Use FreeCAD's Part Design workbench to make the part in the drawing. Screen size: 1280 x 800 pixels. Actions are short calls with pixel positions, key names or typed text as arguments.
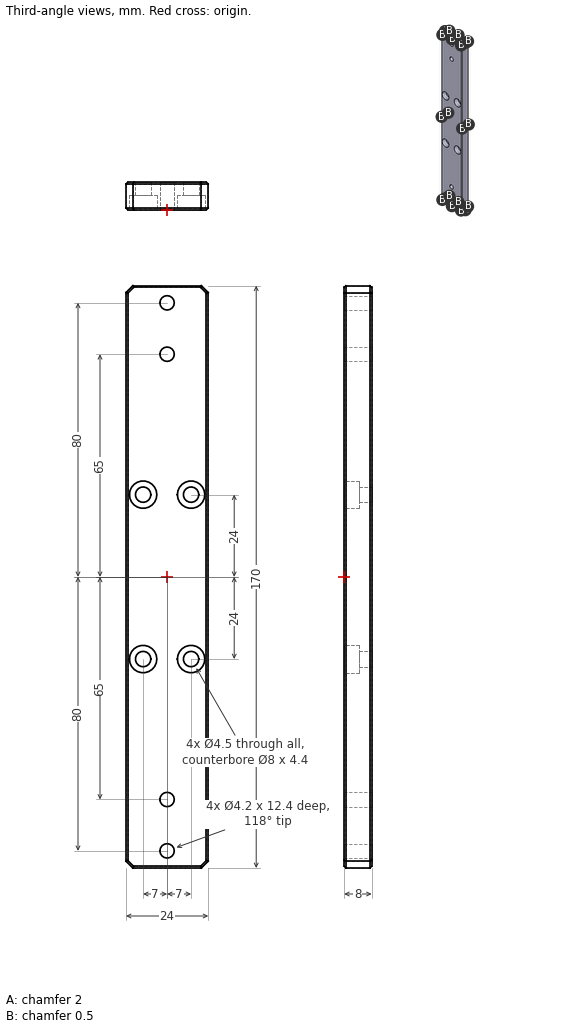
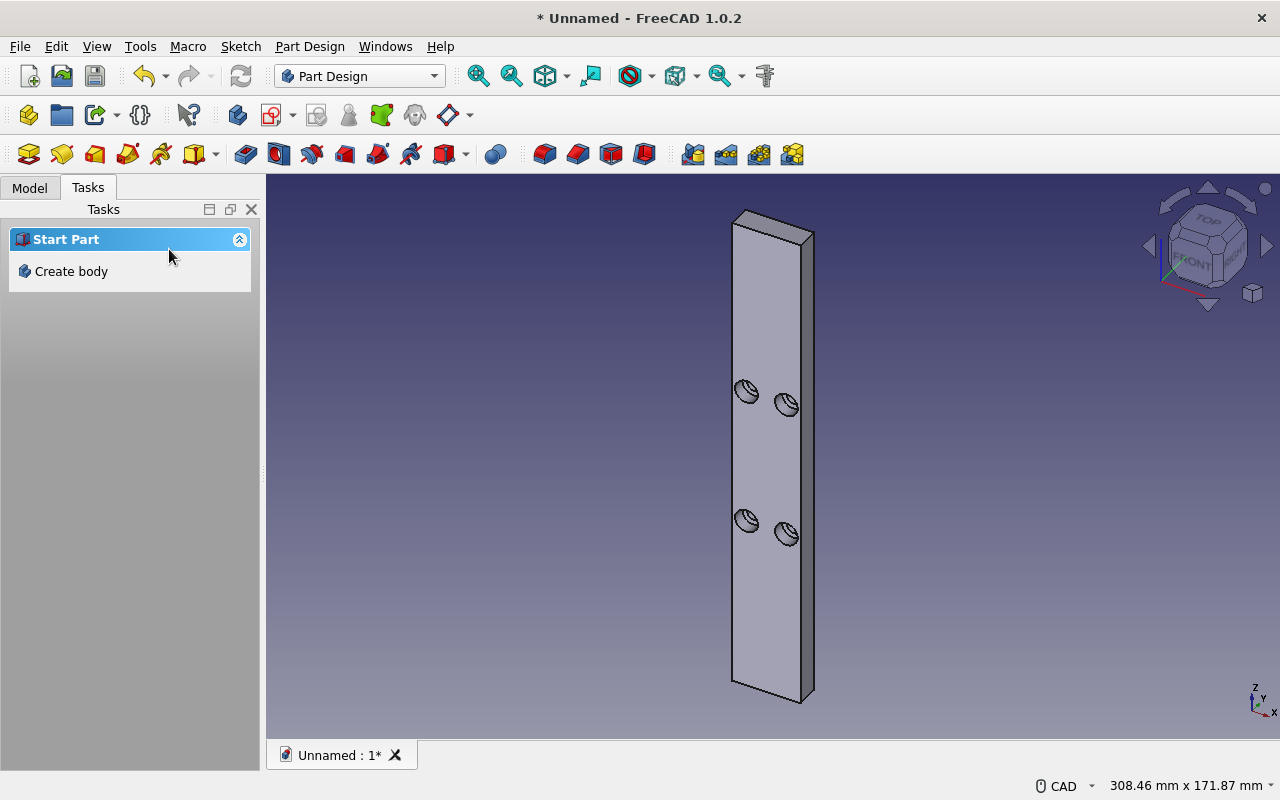
key(4)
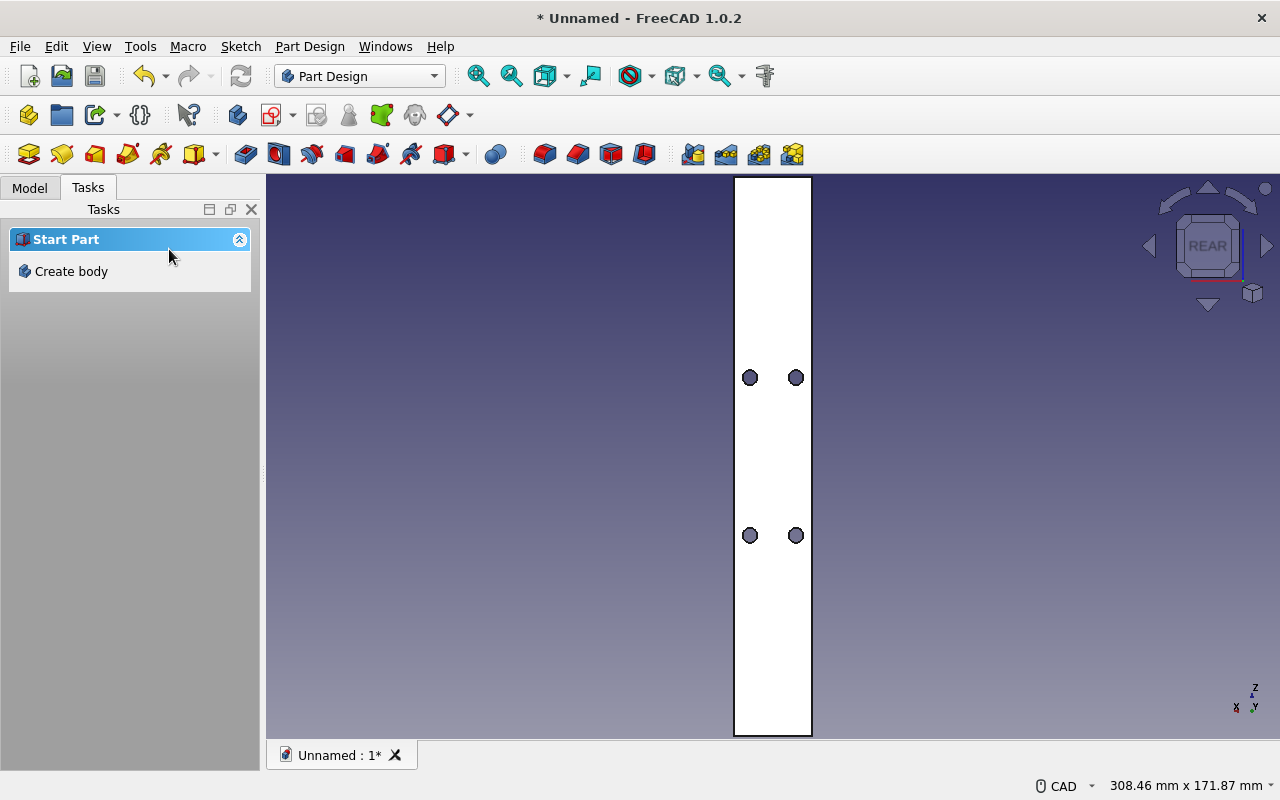
click(773, 216)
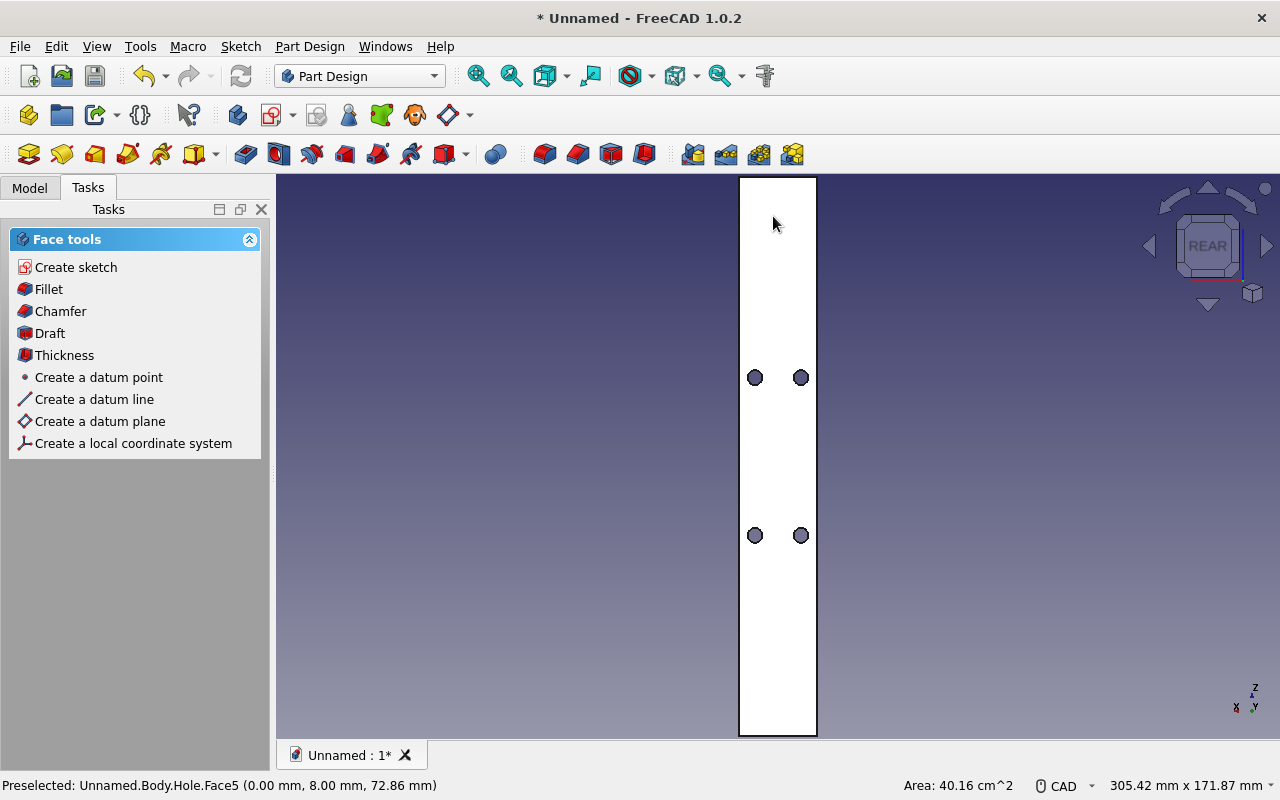
click(270, 116)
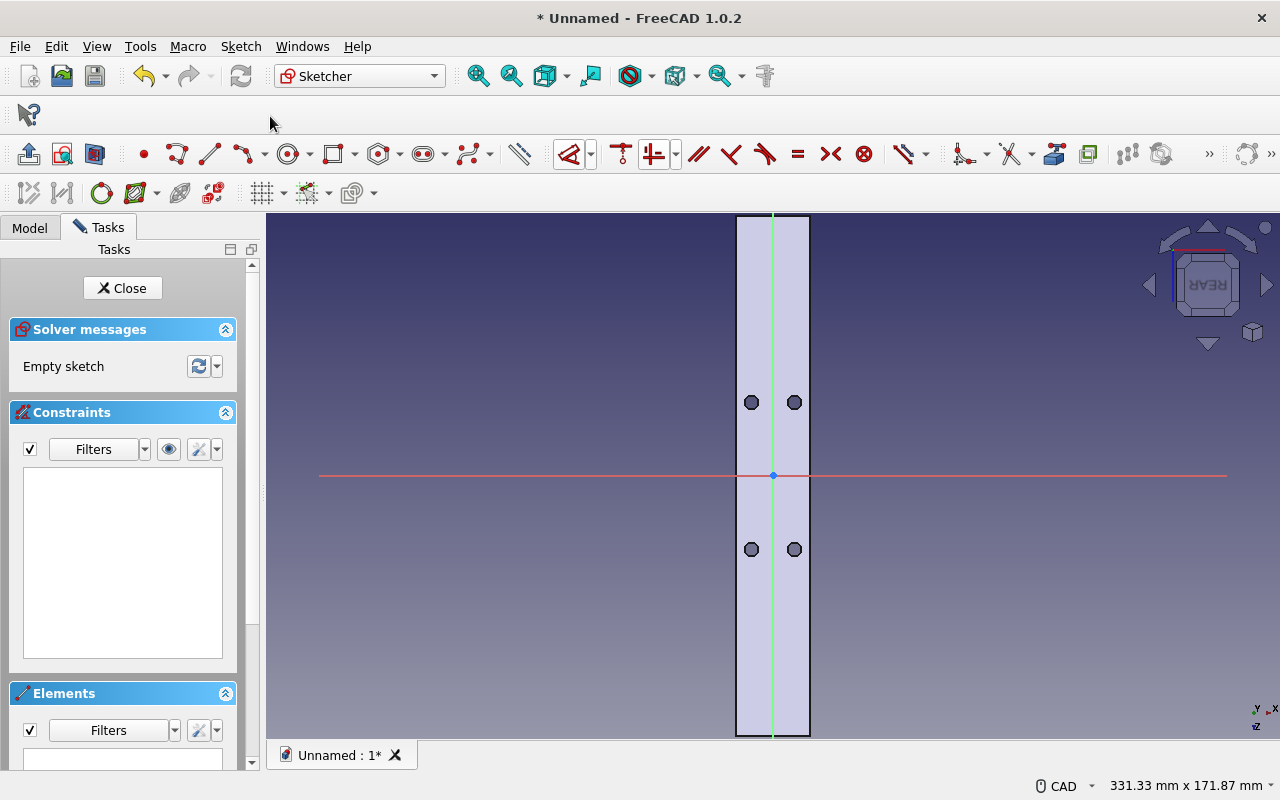
scroll(565, 476, down, 2)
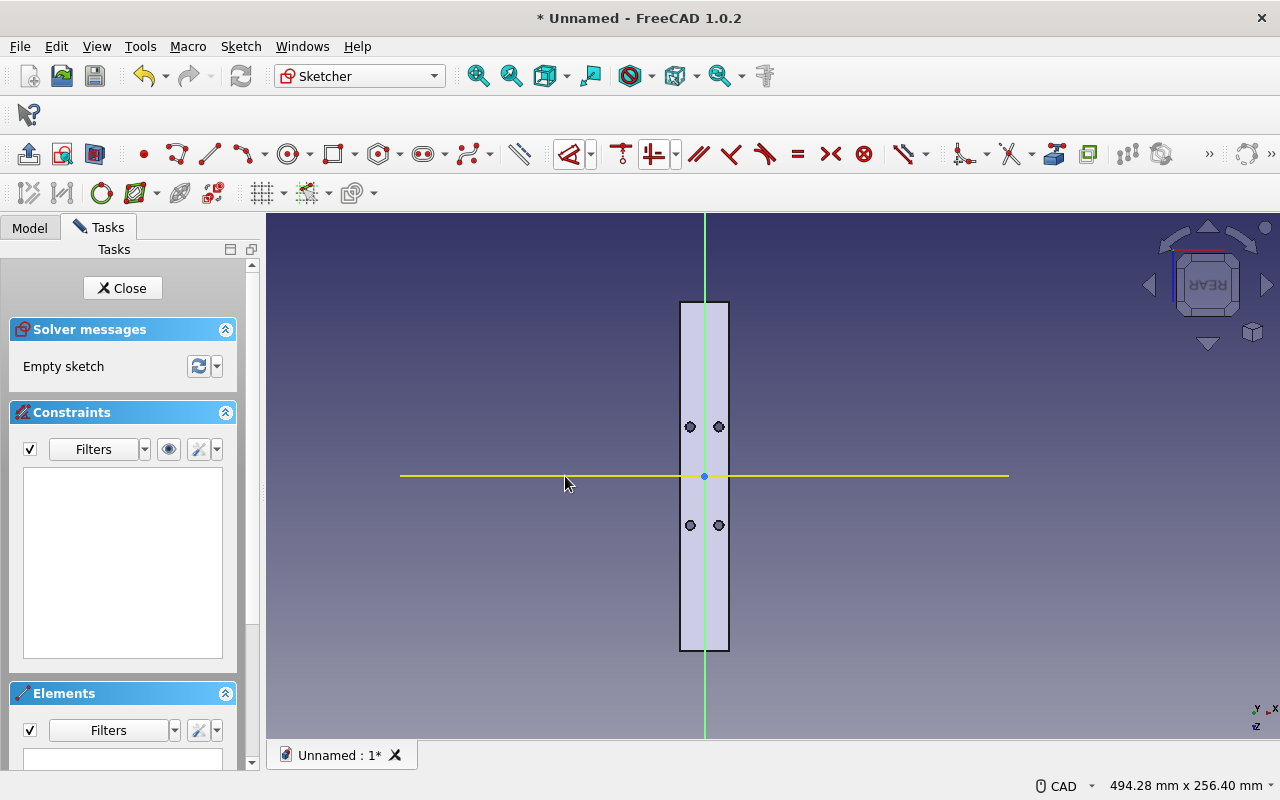
click(288, 154)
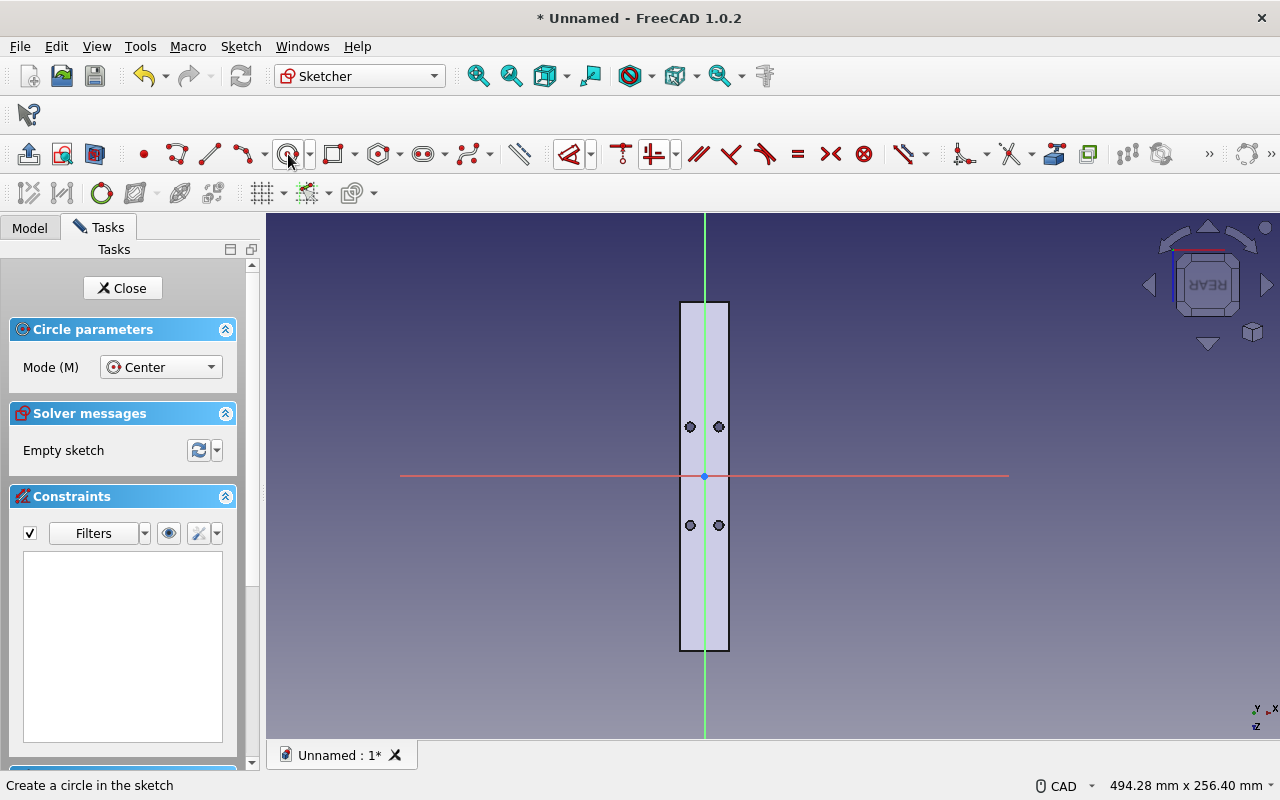
scroll(705, 312, up, 9)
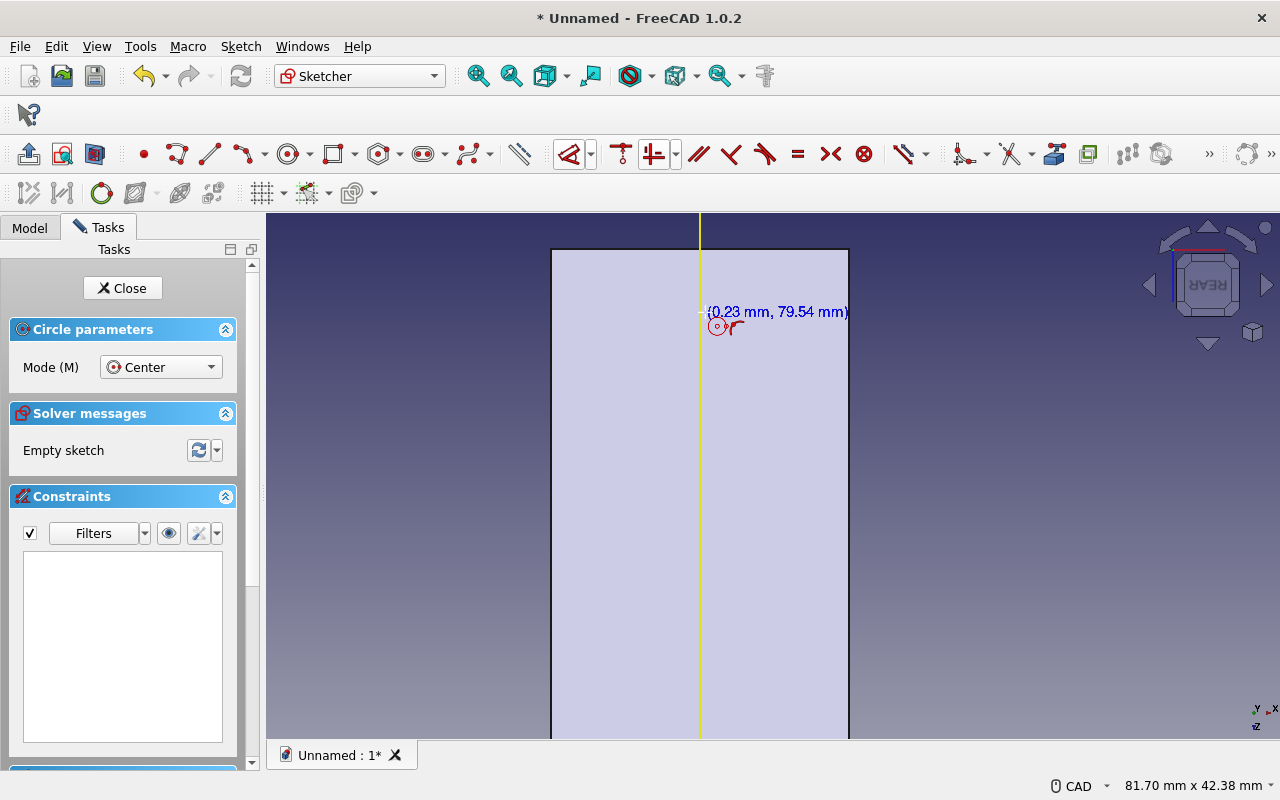
scroll(705, 312, down, 9)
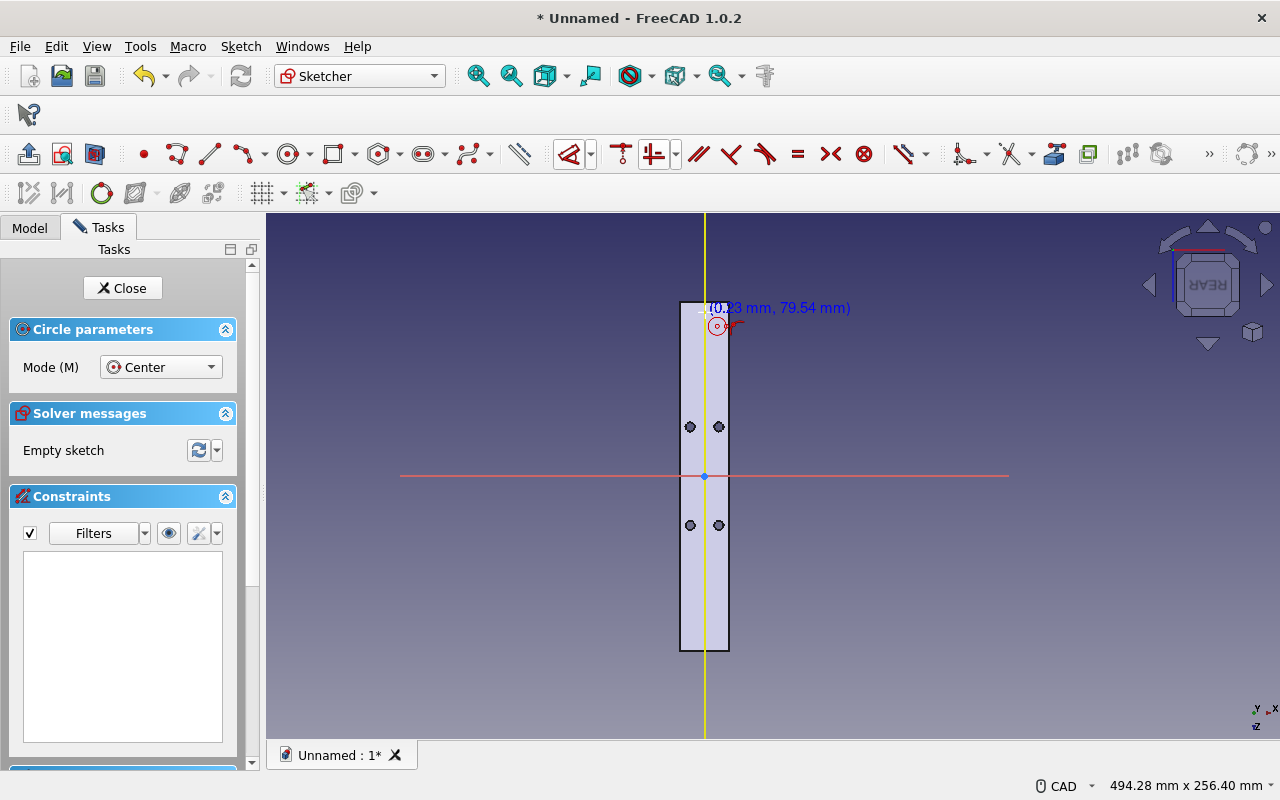
click(705, 312)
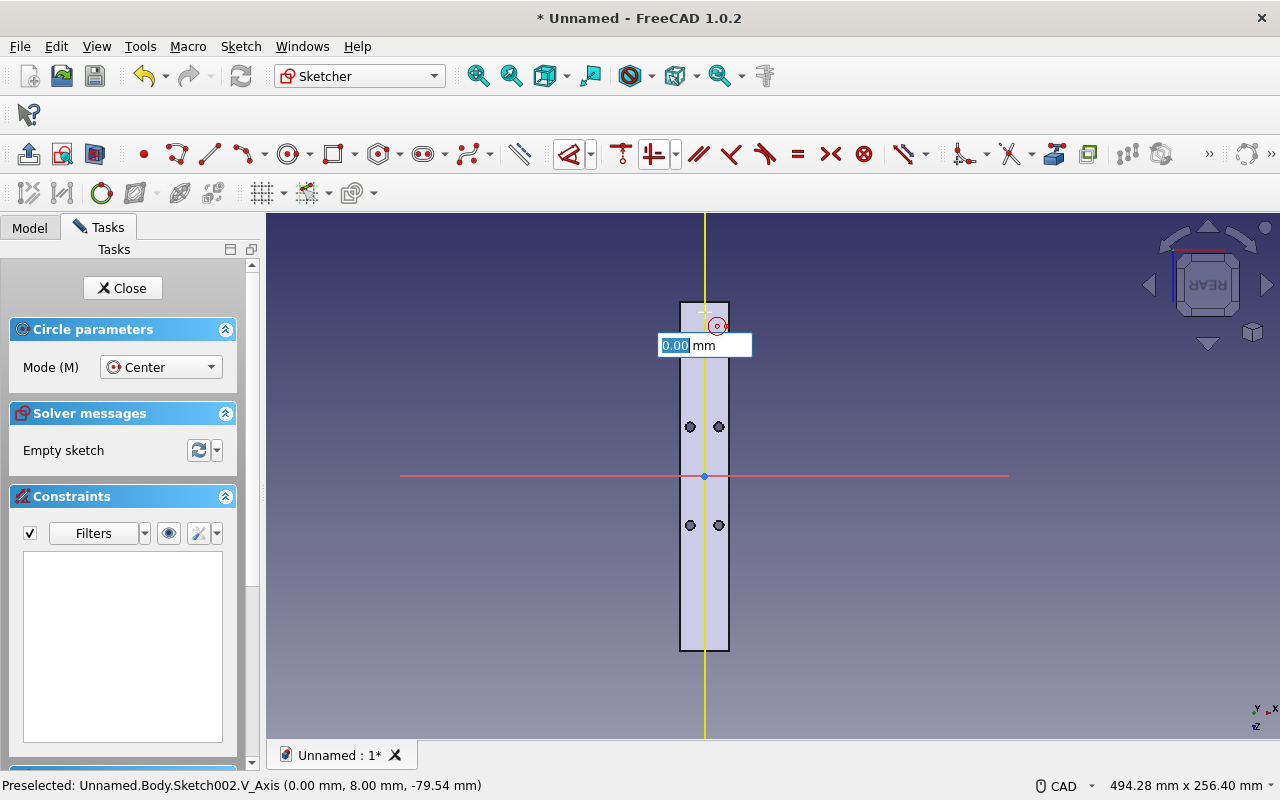
scroll(709, 311, up, 7)
move(706, 309)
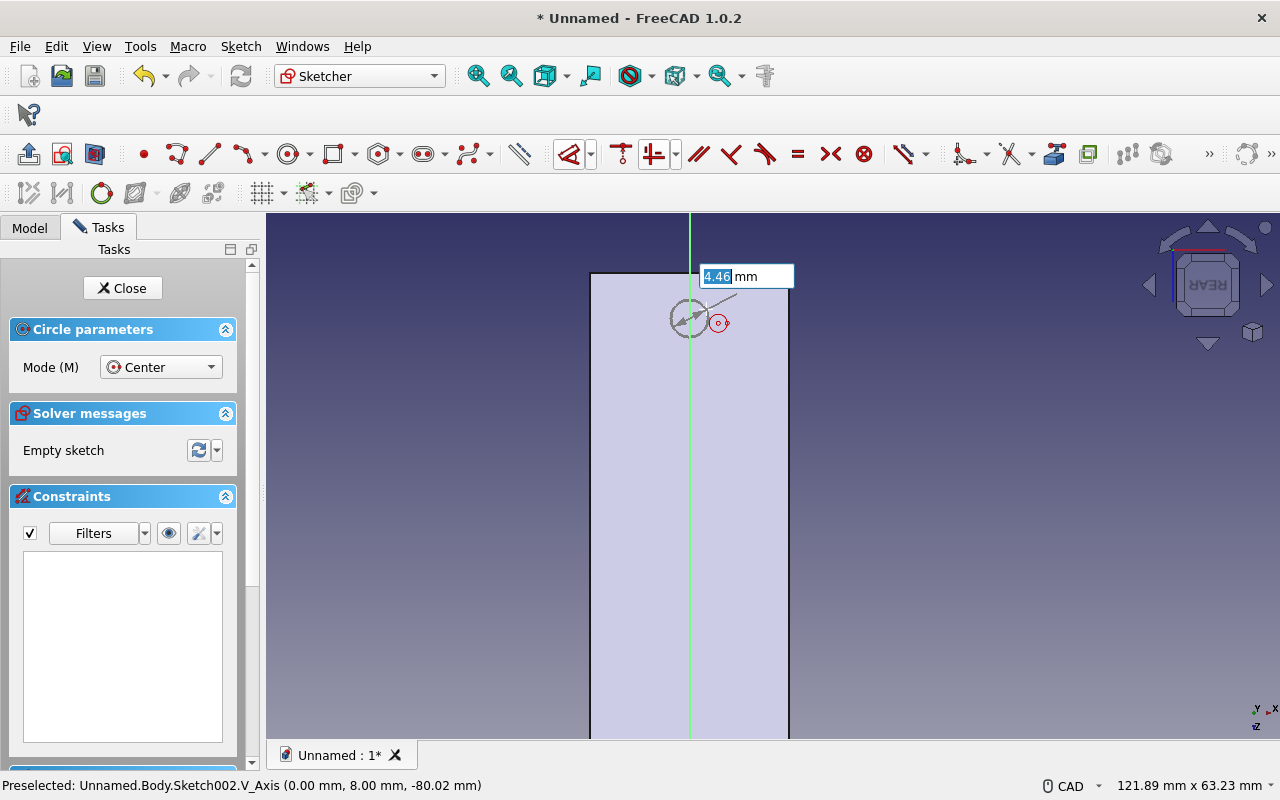
text(4.2)
key(Return)